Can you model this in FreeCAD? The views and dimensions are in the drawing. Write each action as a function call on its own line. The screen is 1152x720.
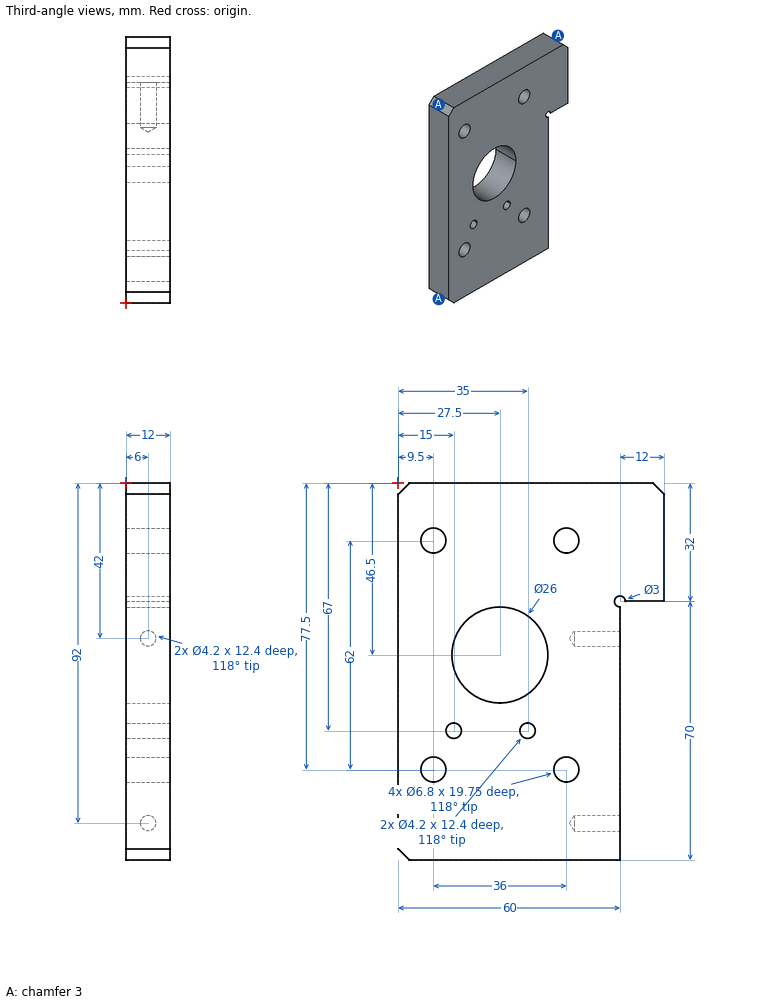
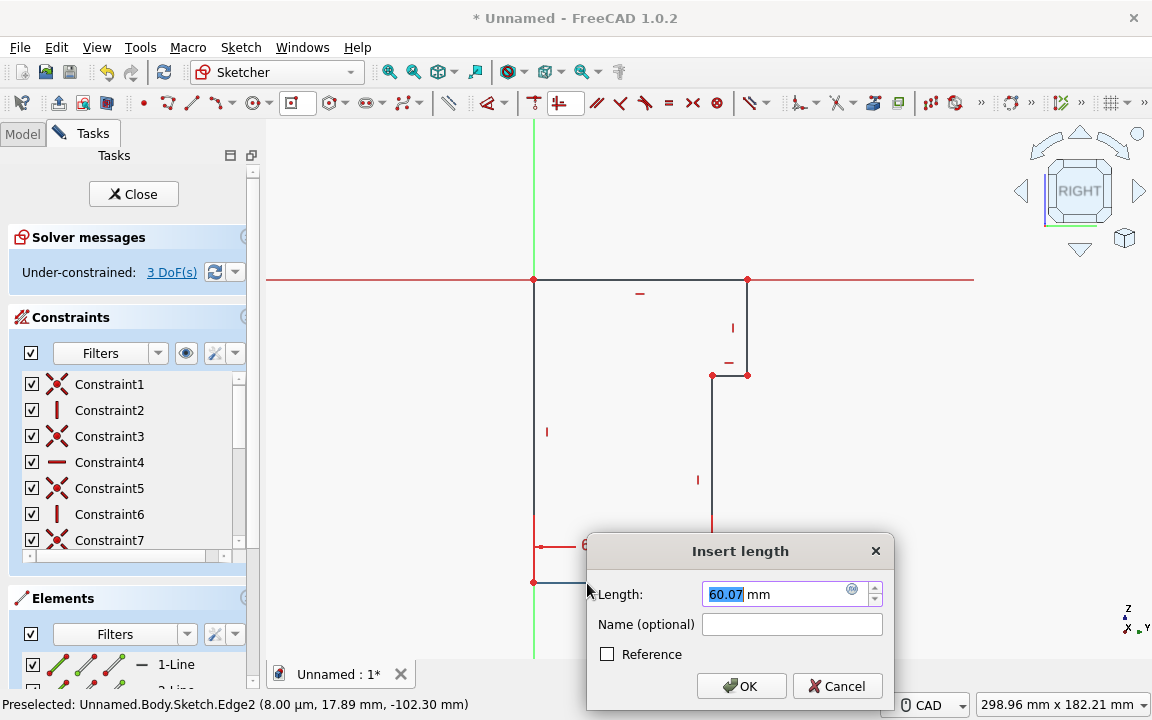
text(60)
key(Return)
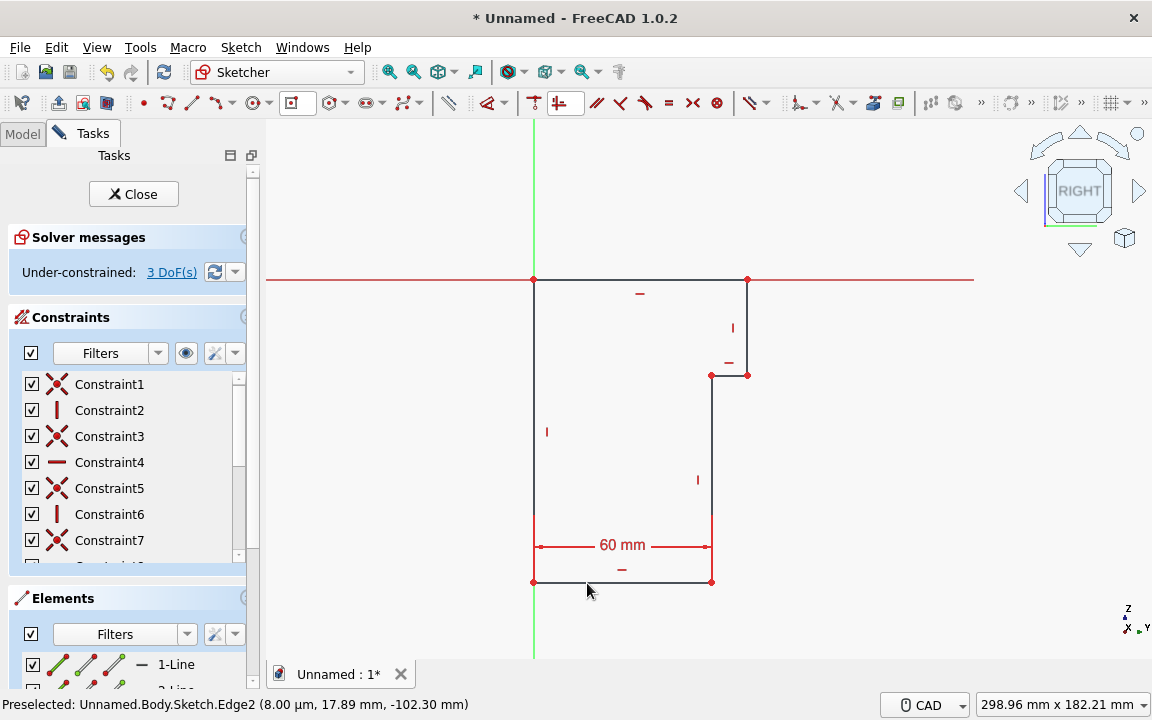
click(712, 521)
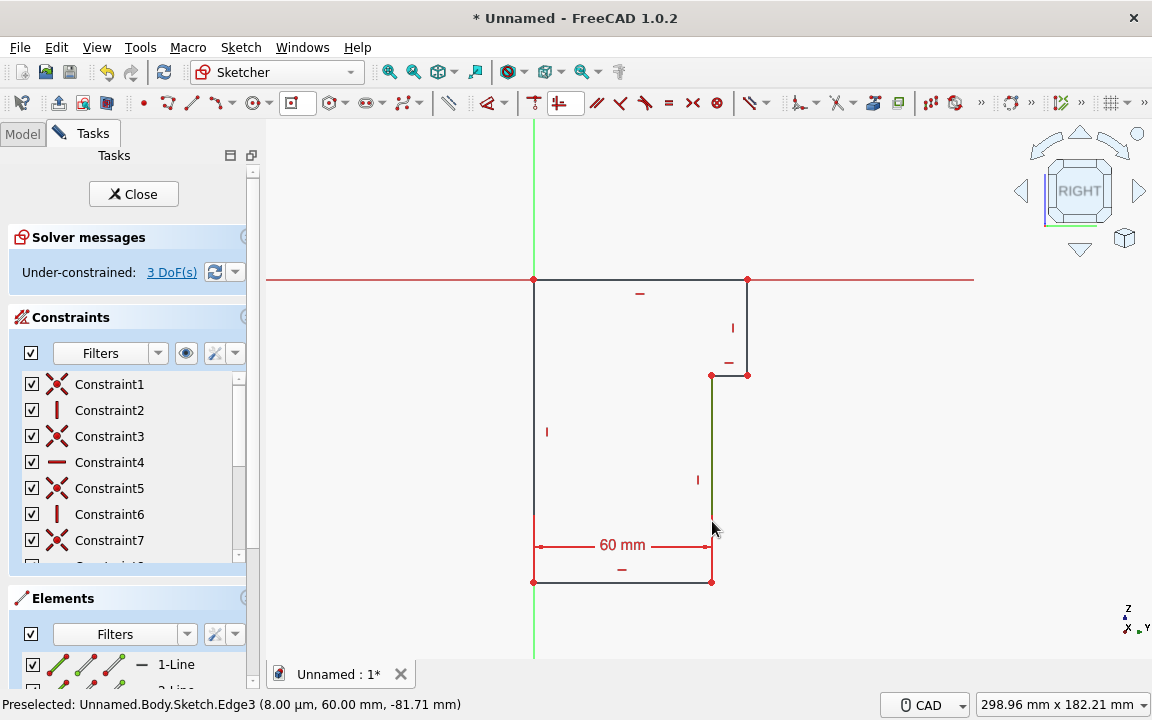
key(i)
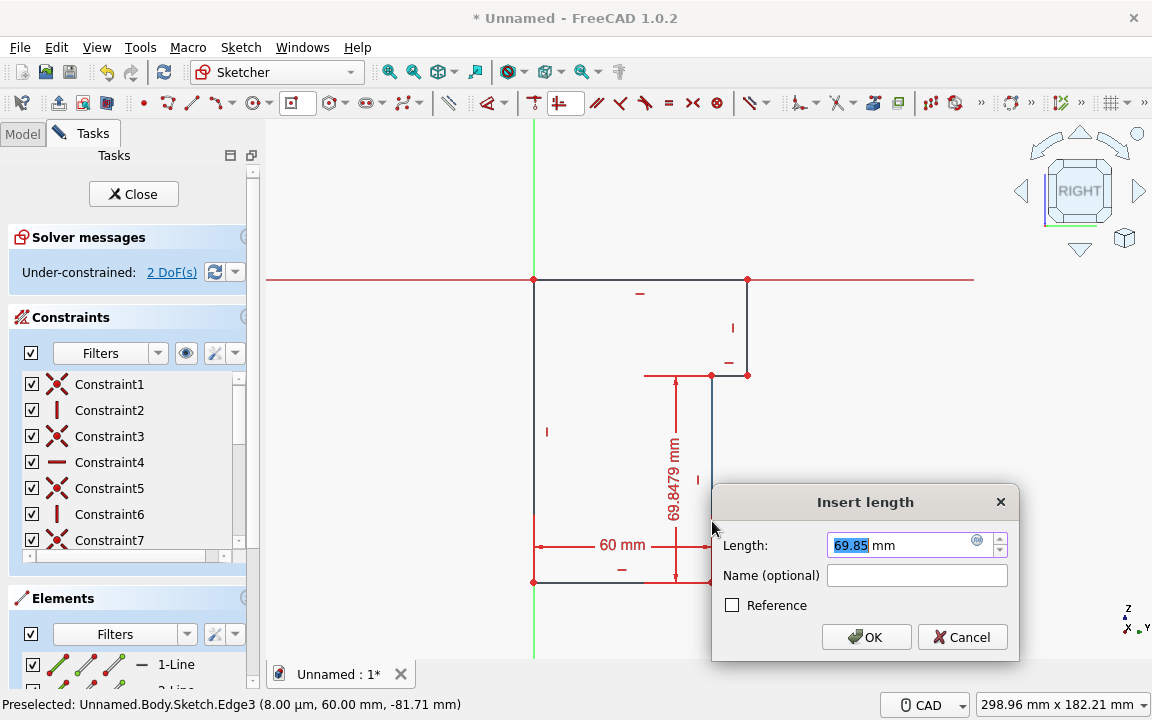
text(70)
key(Return)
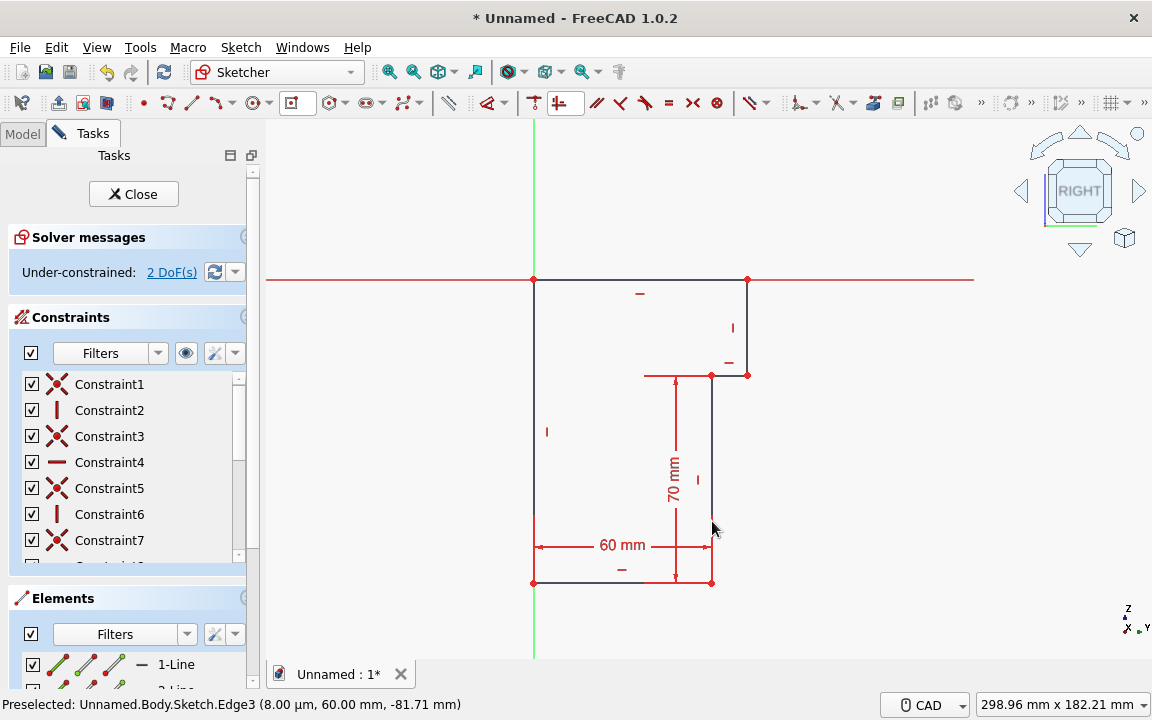
scroll(722, 376, up, 2)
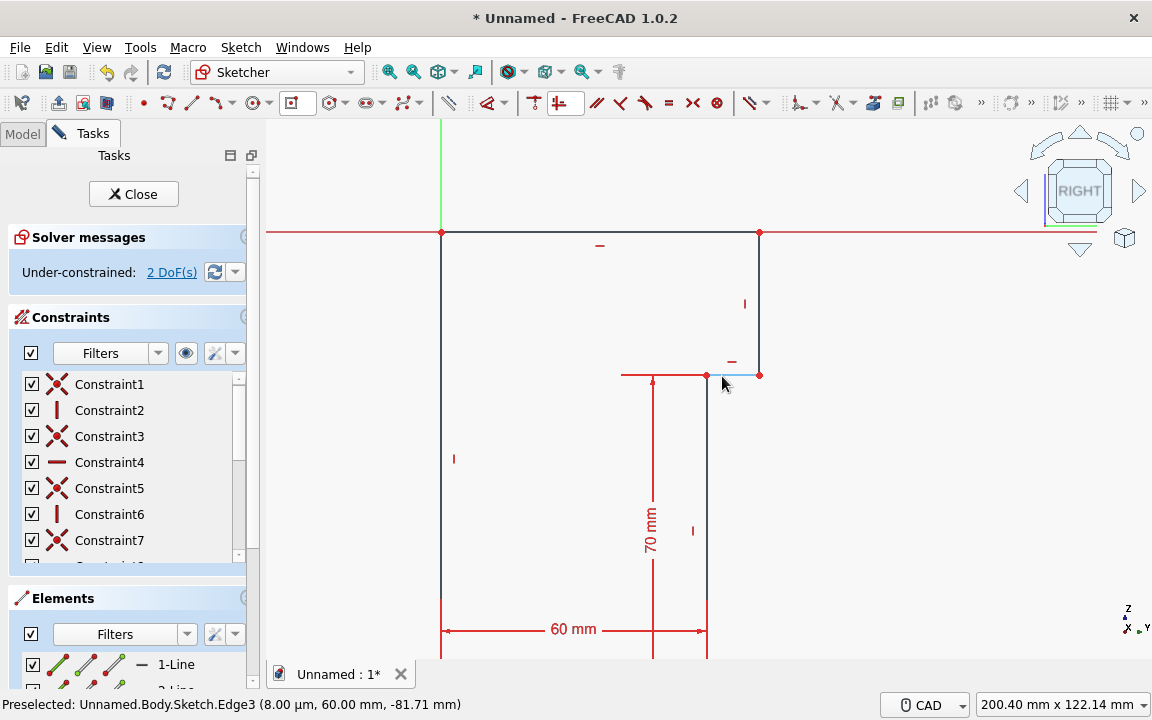
click(722, 375)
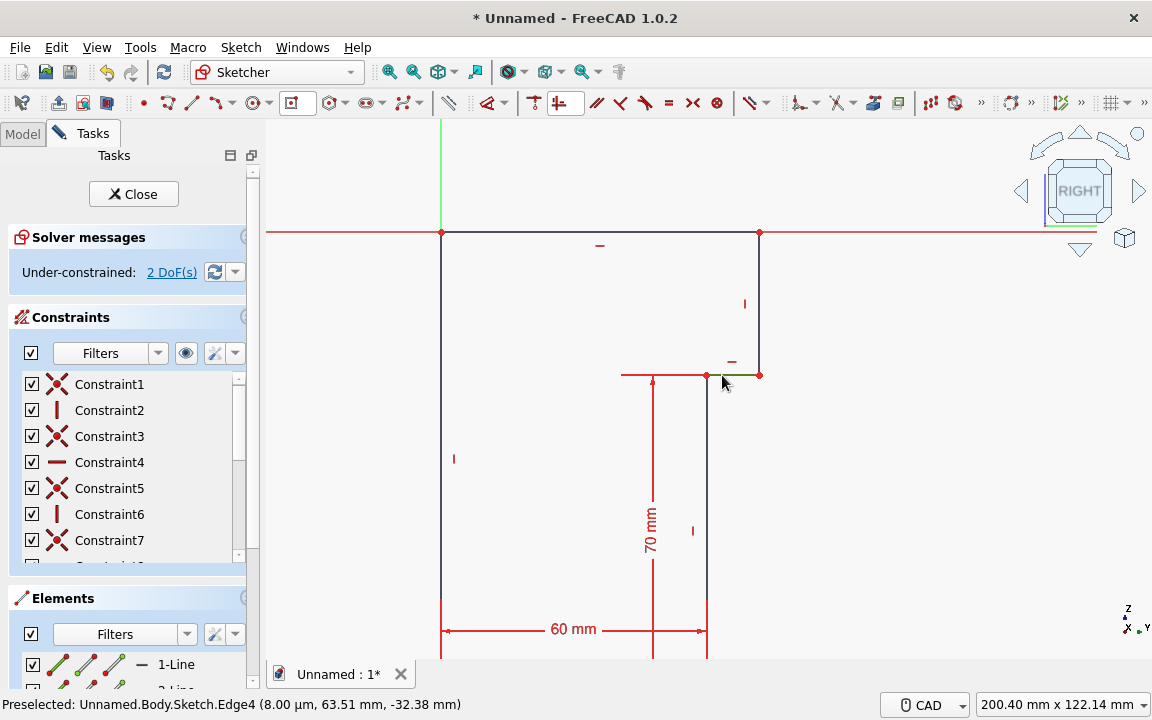
key(l)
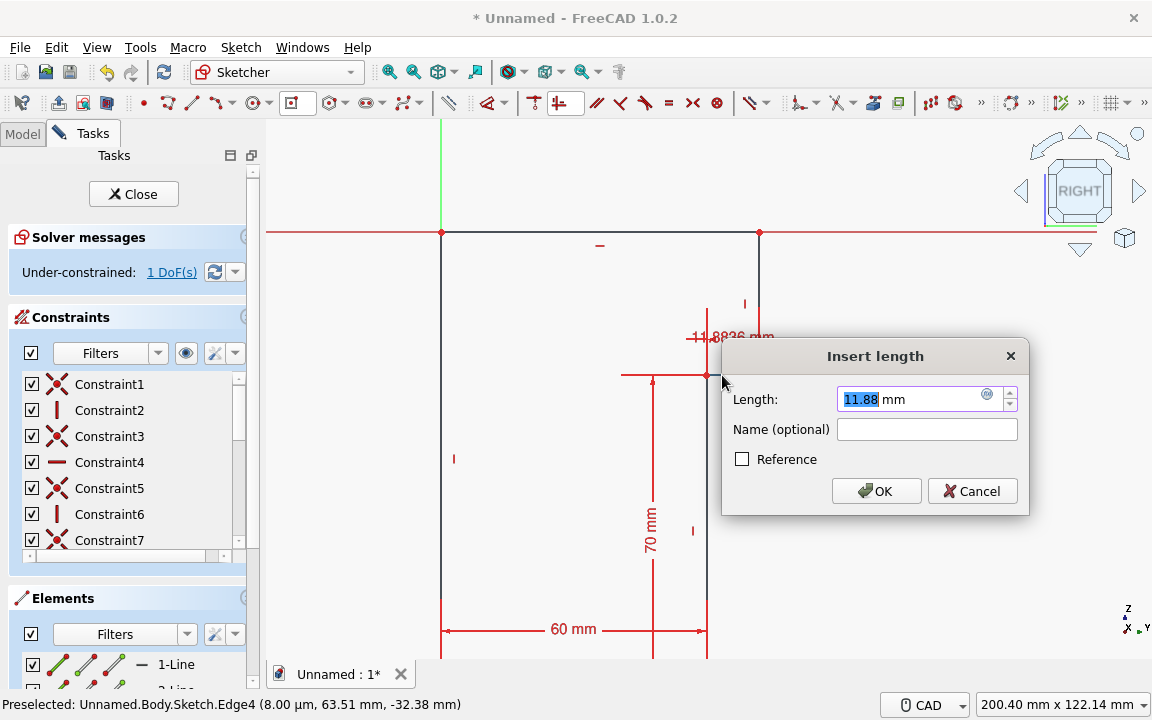
text(12)
key(Return)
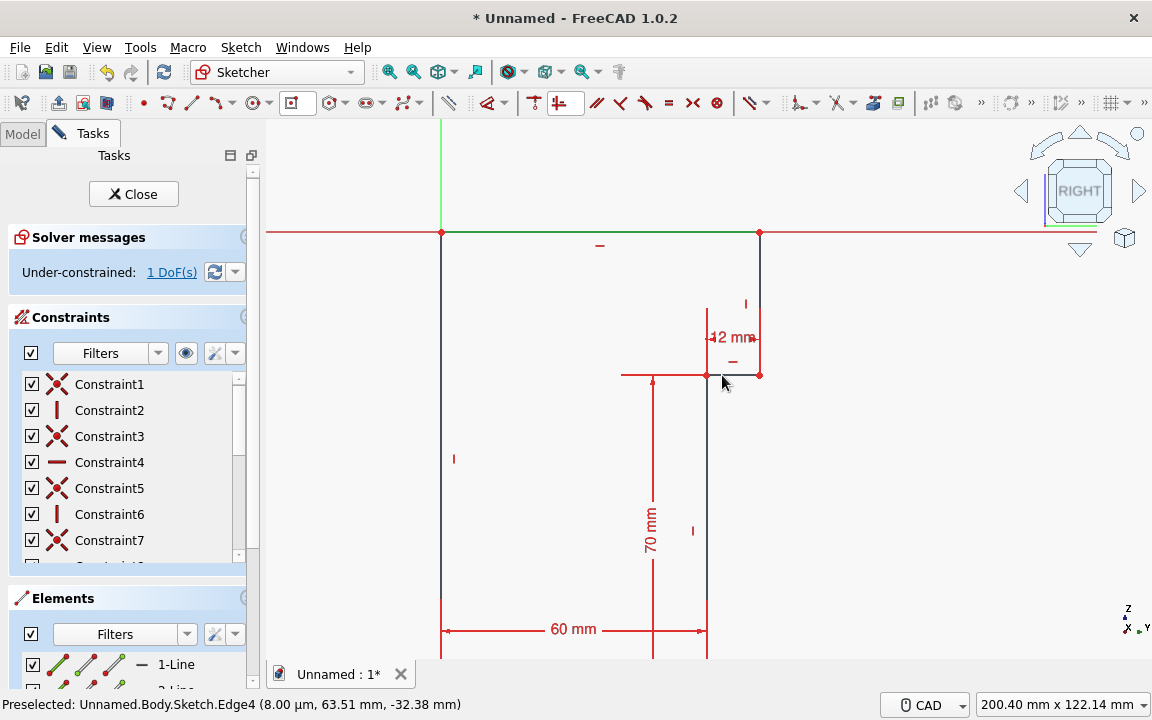
click(760, 333)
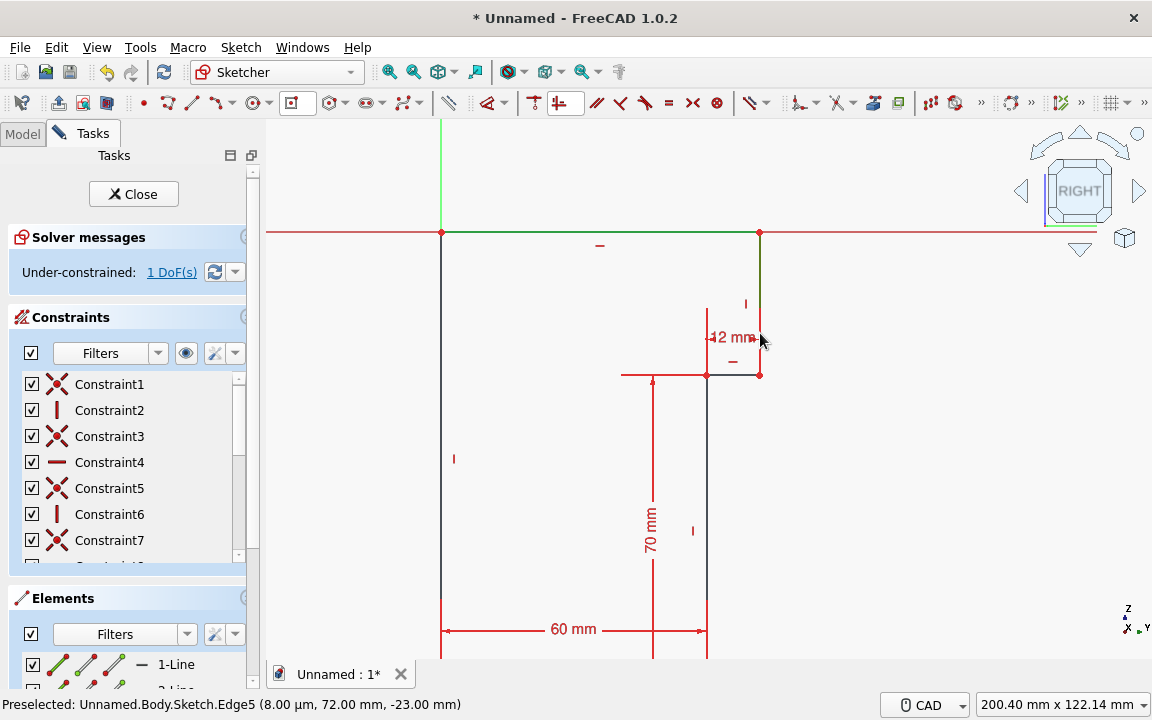
key(i)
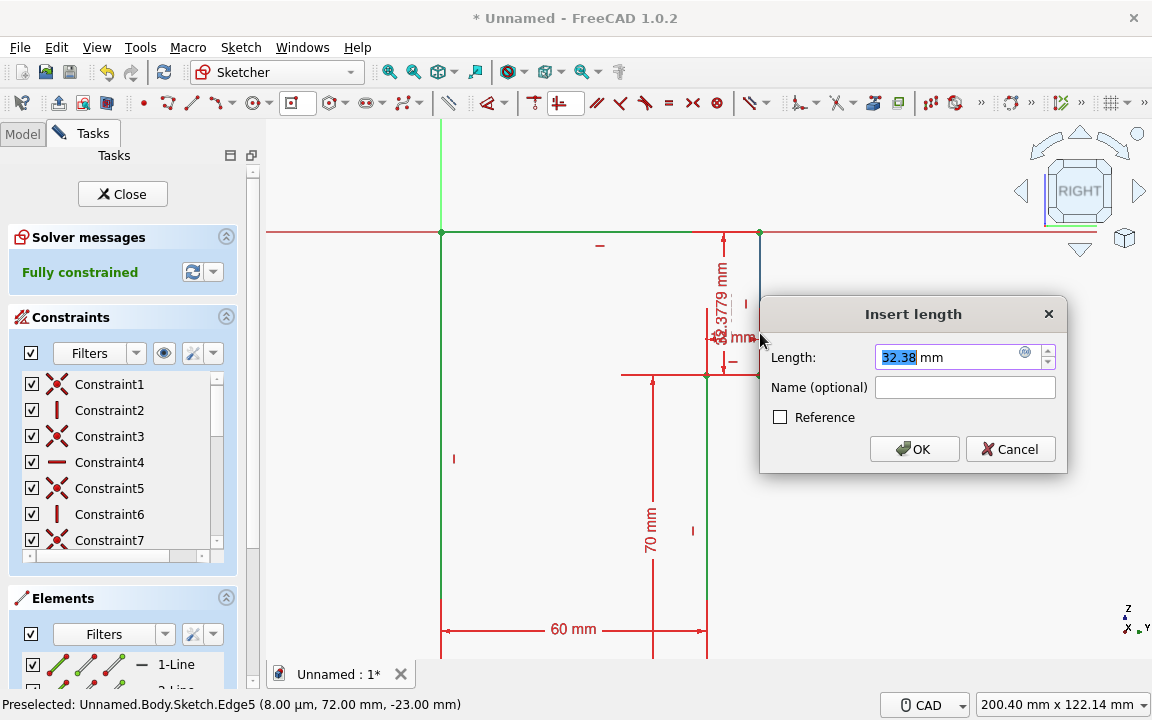
text(32)
key(Return)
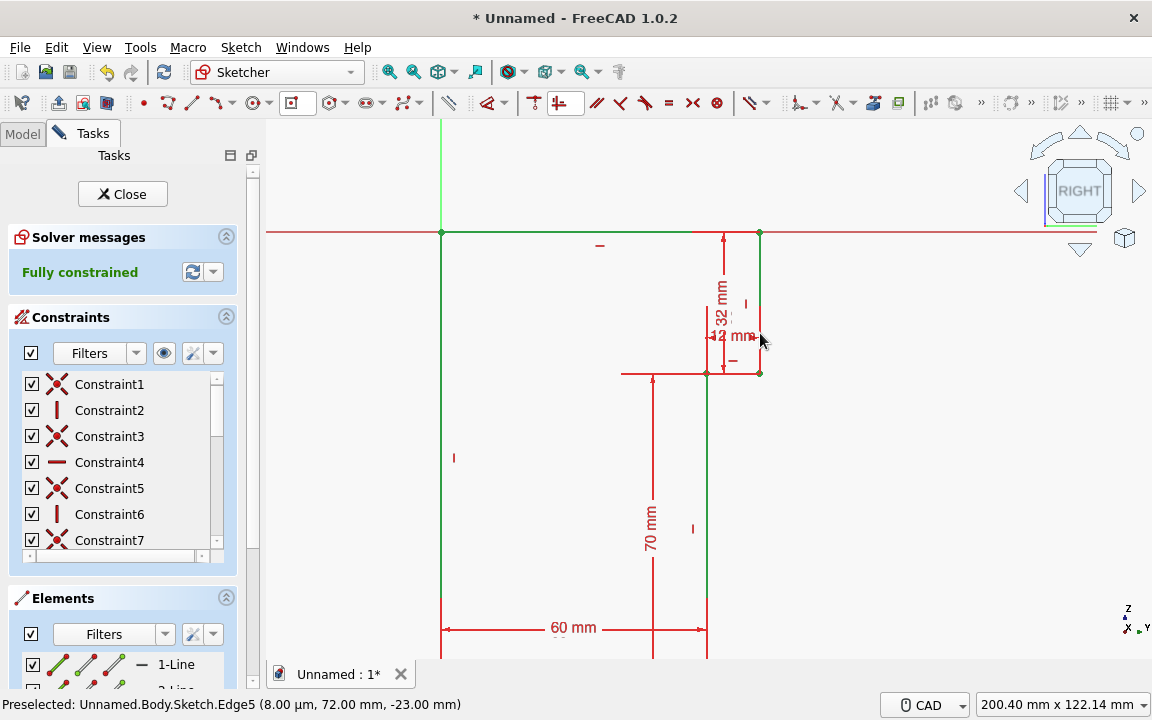
click(123, 194)